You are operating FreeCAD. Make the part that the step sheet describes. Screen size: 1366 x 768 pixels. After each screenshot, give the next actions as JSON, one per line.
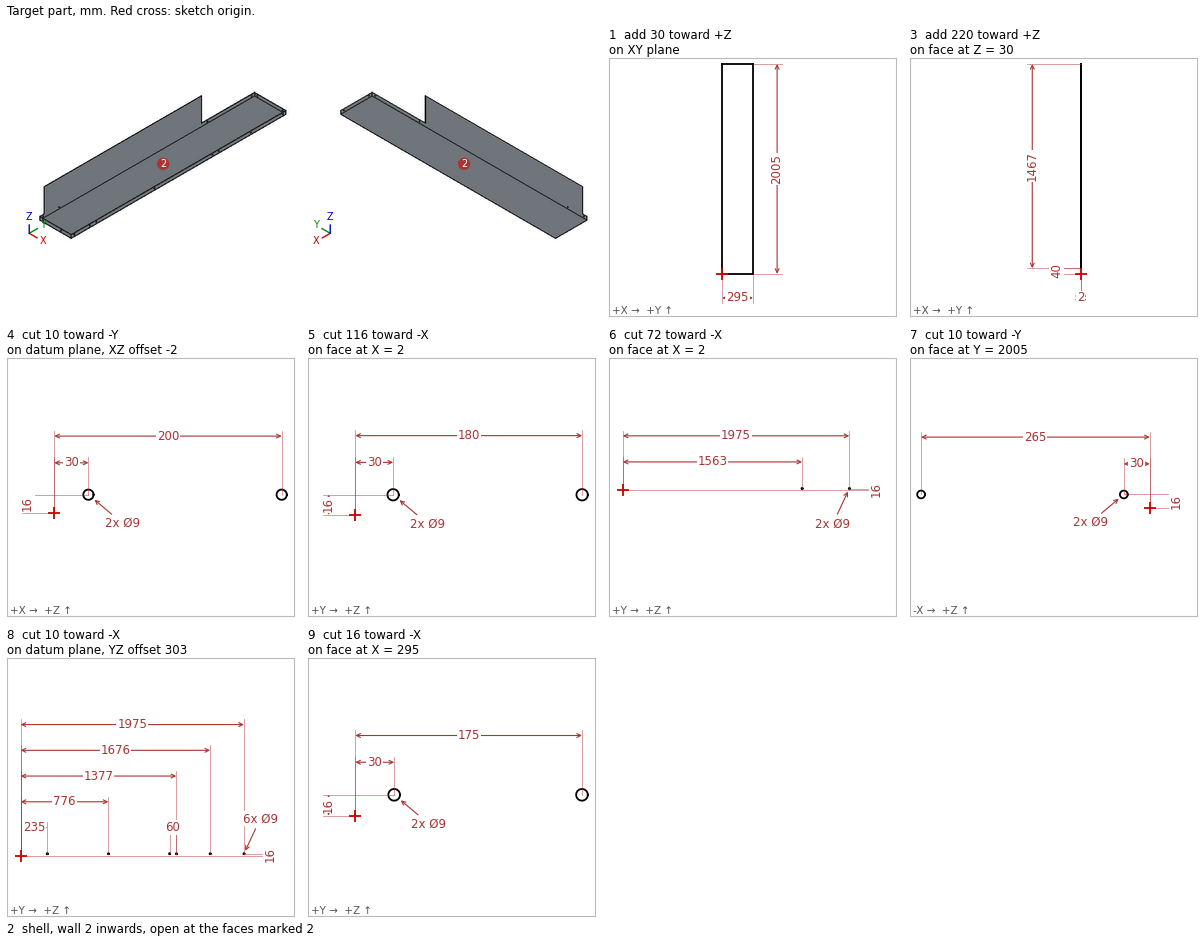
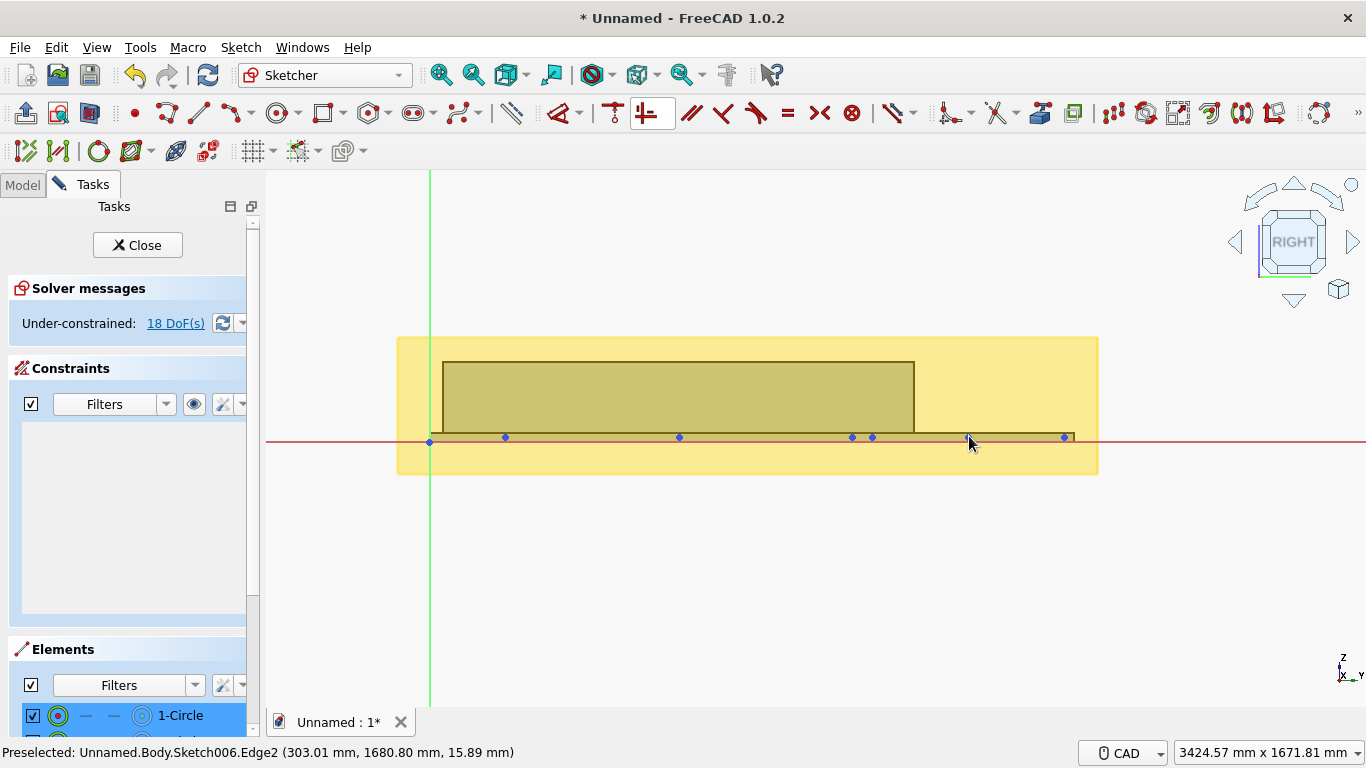
{"action": "scroll", "coordinate": [873, 436], "scroll_direction": "up", "scroll_amount": 11}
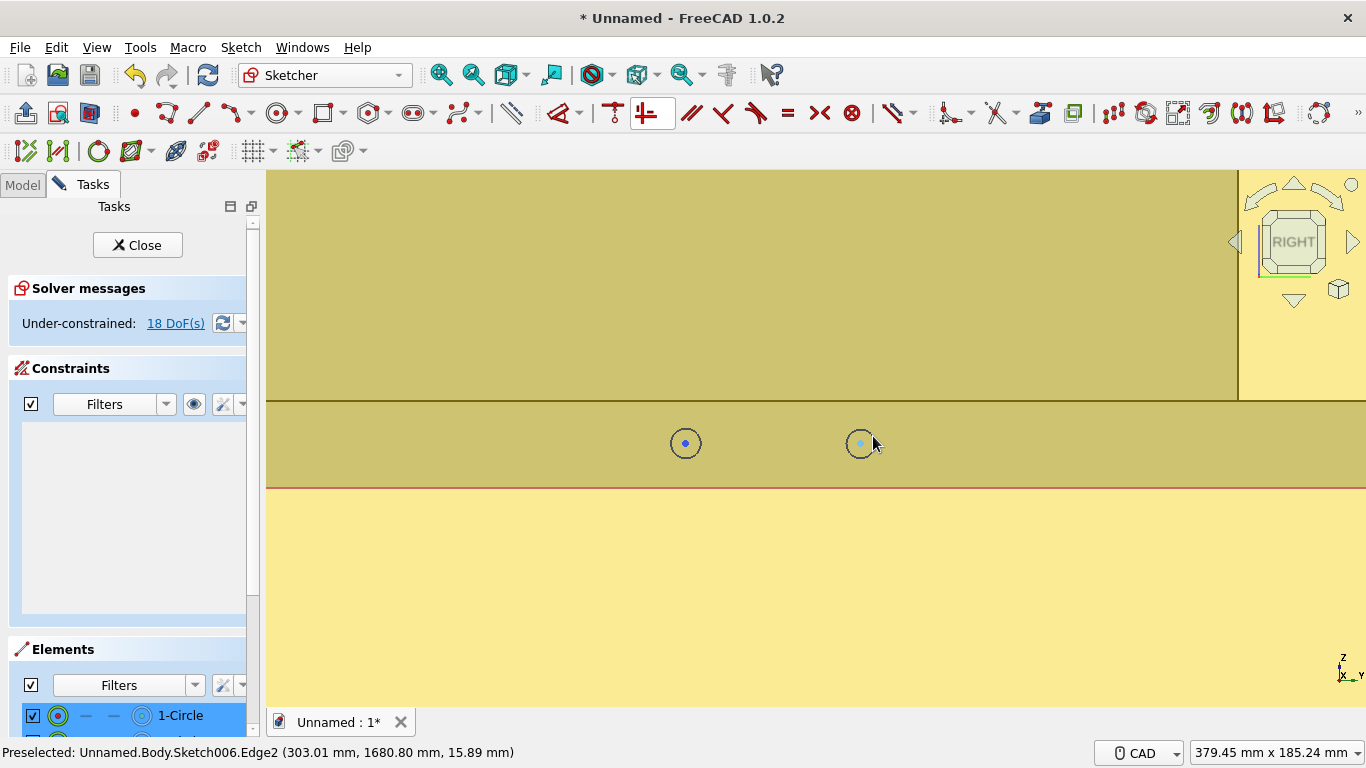
{"action": "left_click", "coordinate": [871, 434]}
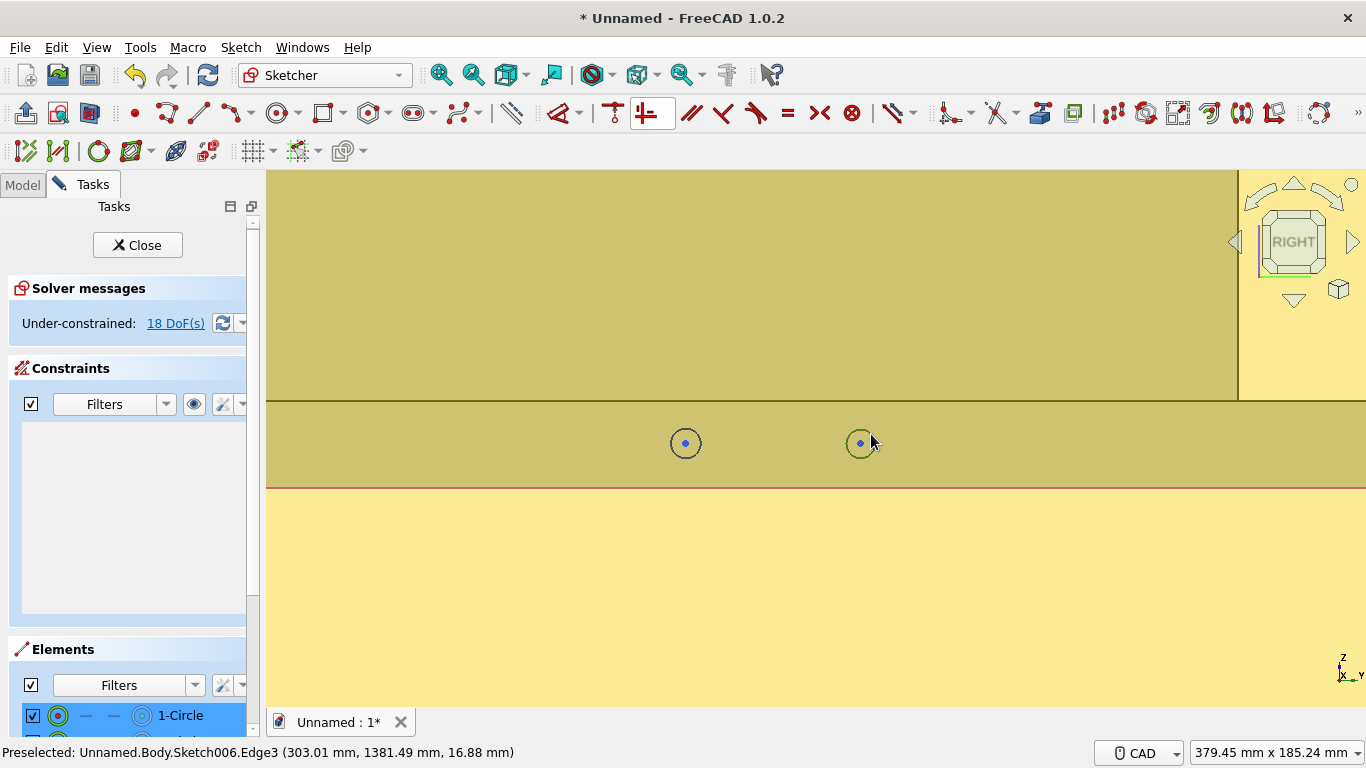
{"action": "left_click", "coordinate": [696, 433]}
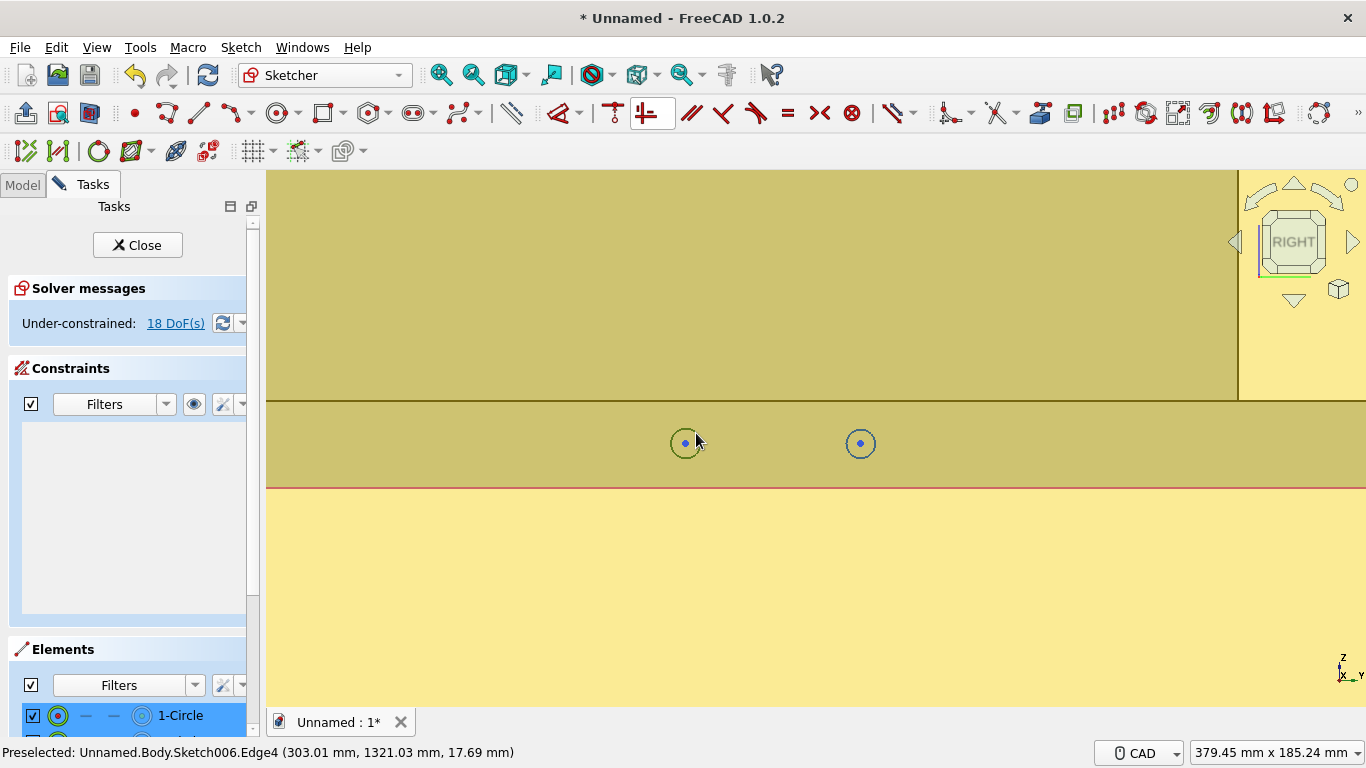
{"action": "scroll", "coordinate": [873, 436], "scroll_direction": "down", "scroll_amount": 11}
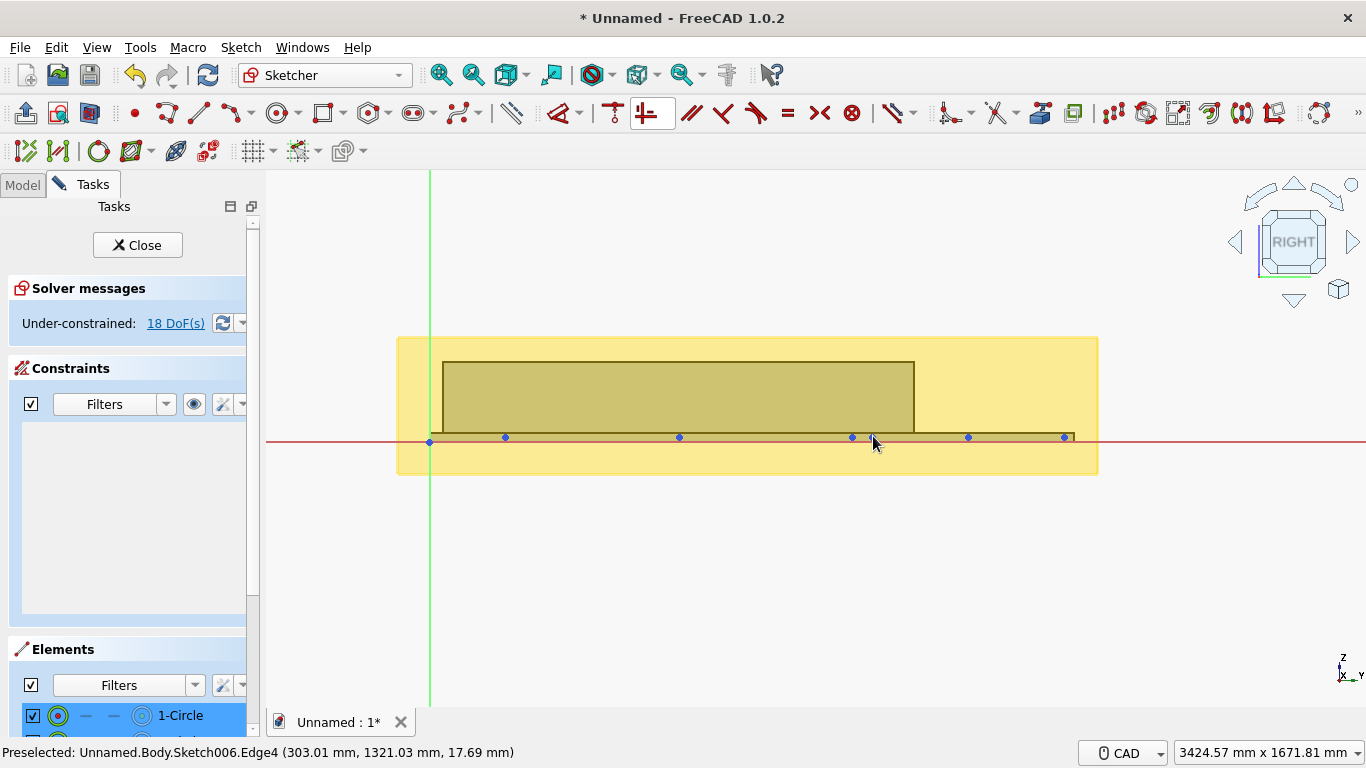
{"action": "scroll", "coordinate": [680, 436], "scroll_direction": "up", "scroll_amount": 11}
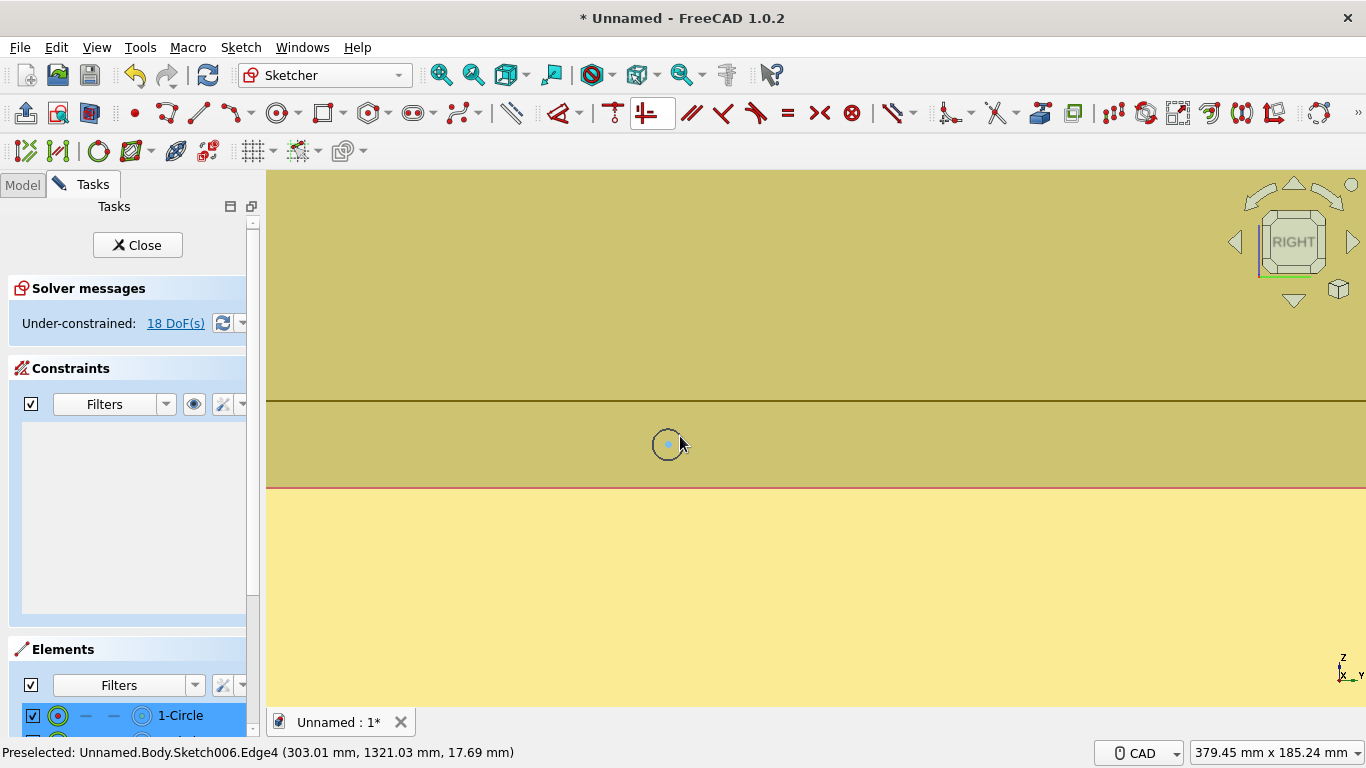
{"action": "left_click", "coordinate": [679, 434]}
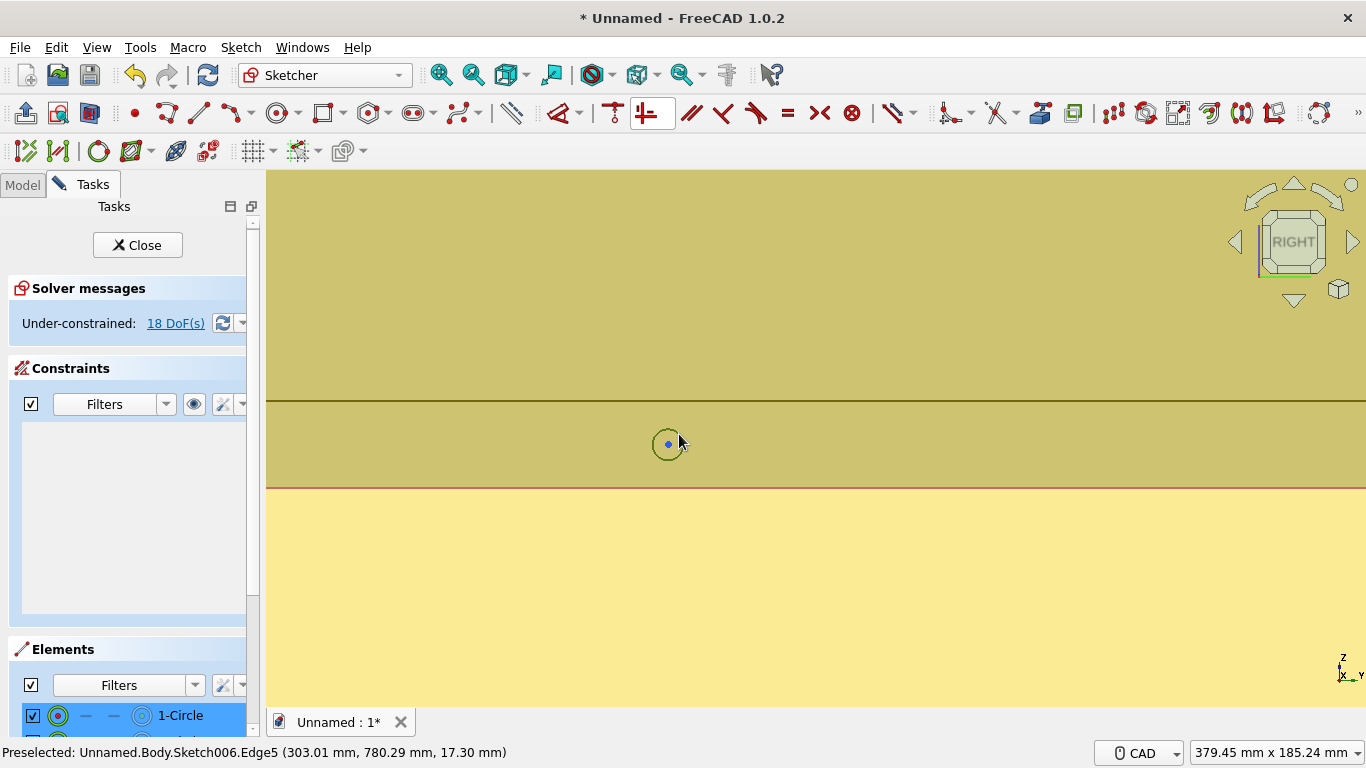
{"action": "scroll", "coordinate": [680, 436], "scroll_direction": "down", "scroll_amount": 11}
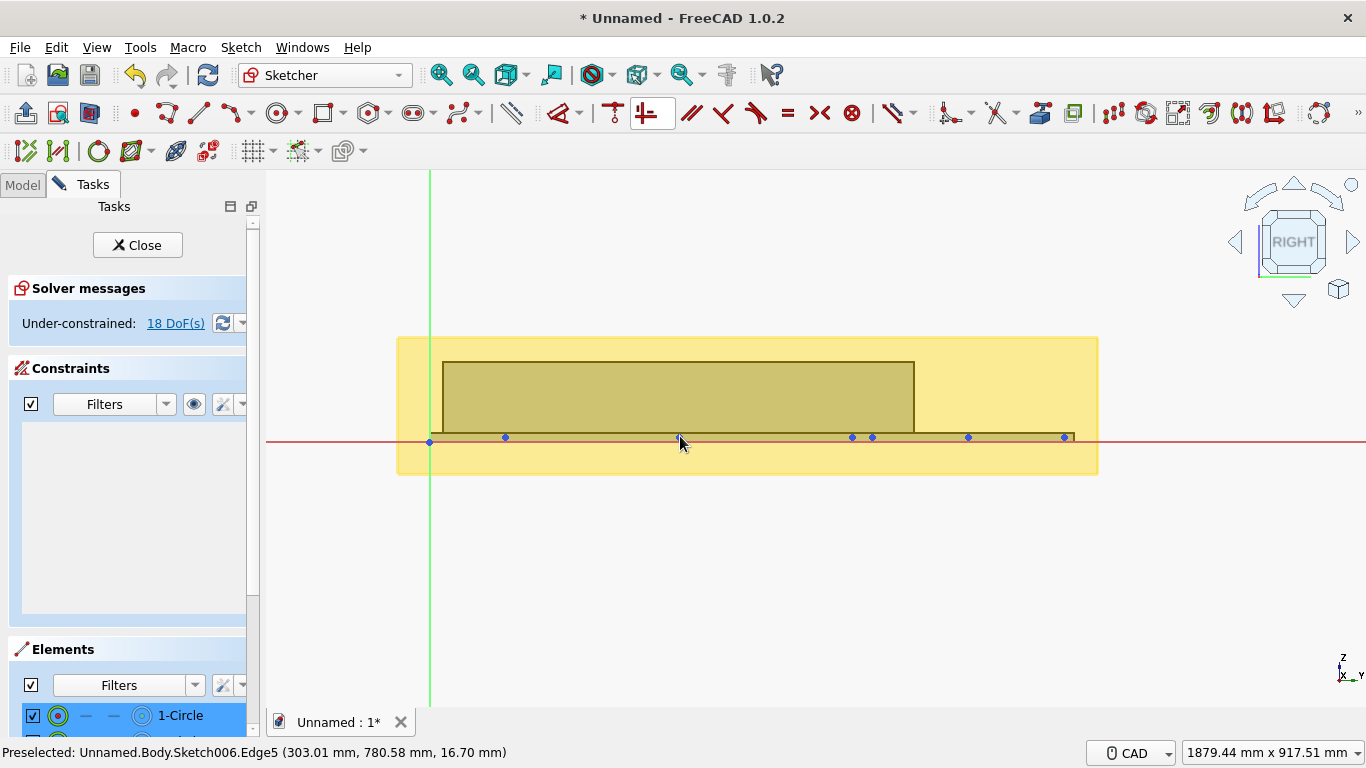
{"action": "scroll", "coordinate": [506, 436], "scroll_direction": "up", "scroll_amount": 11}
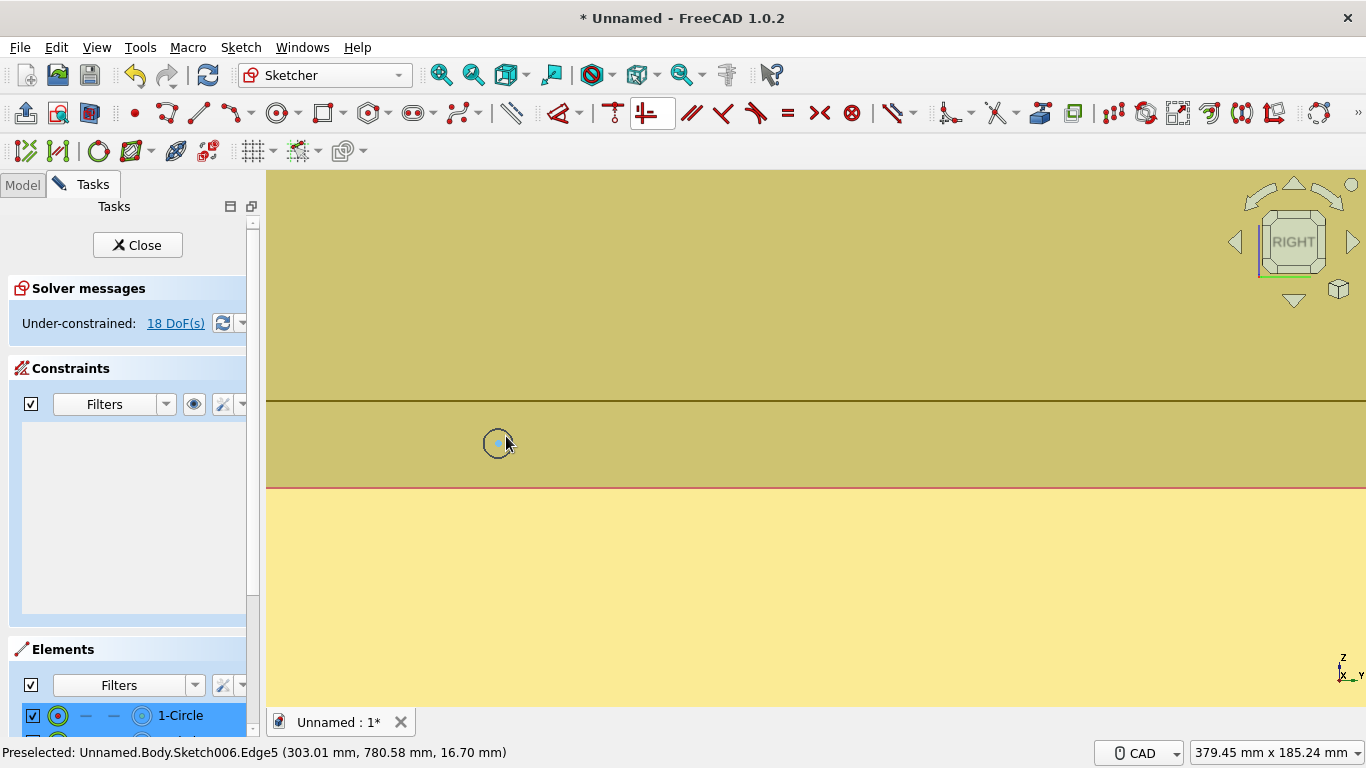
{"action": "left_click", "coordinate": [508, 433]}